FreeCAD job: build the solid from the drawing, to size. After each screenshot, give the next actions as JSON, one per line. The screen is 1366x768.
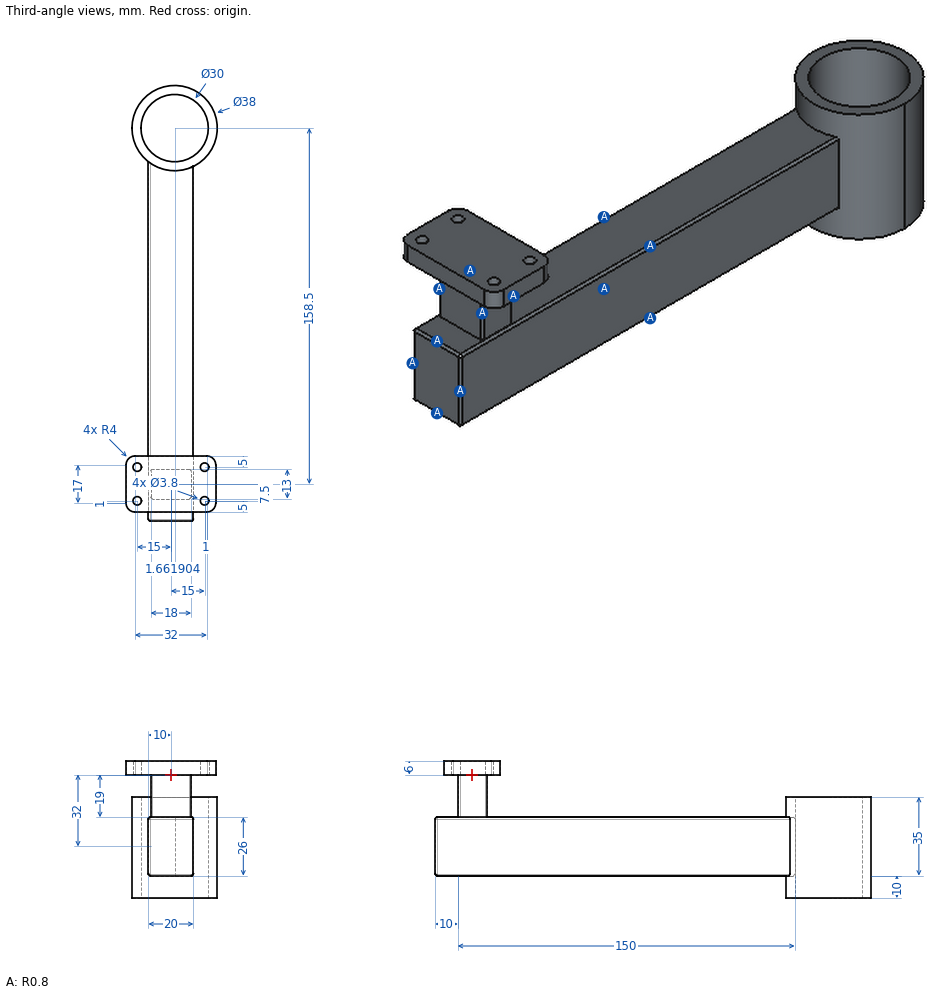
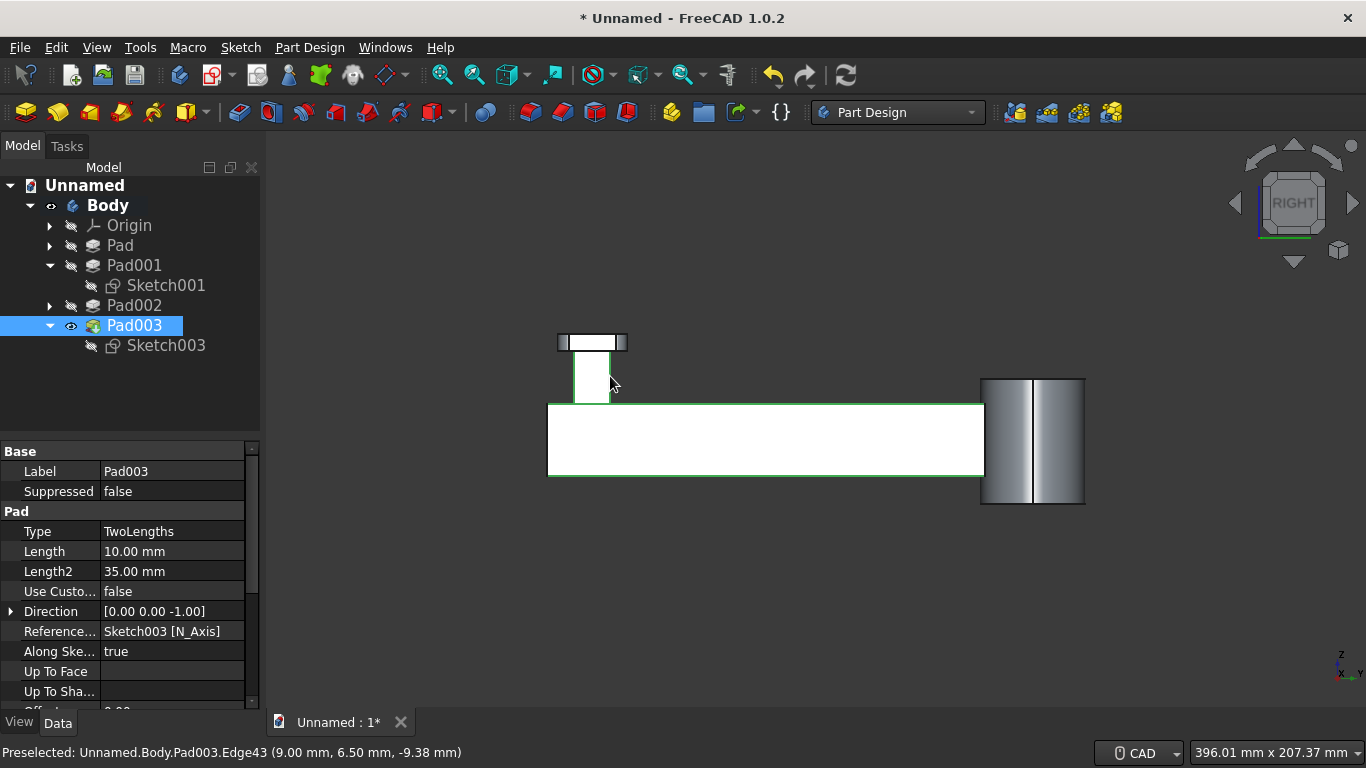
{"action": "key", "text": "5"}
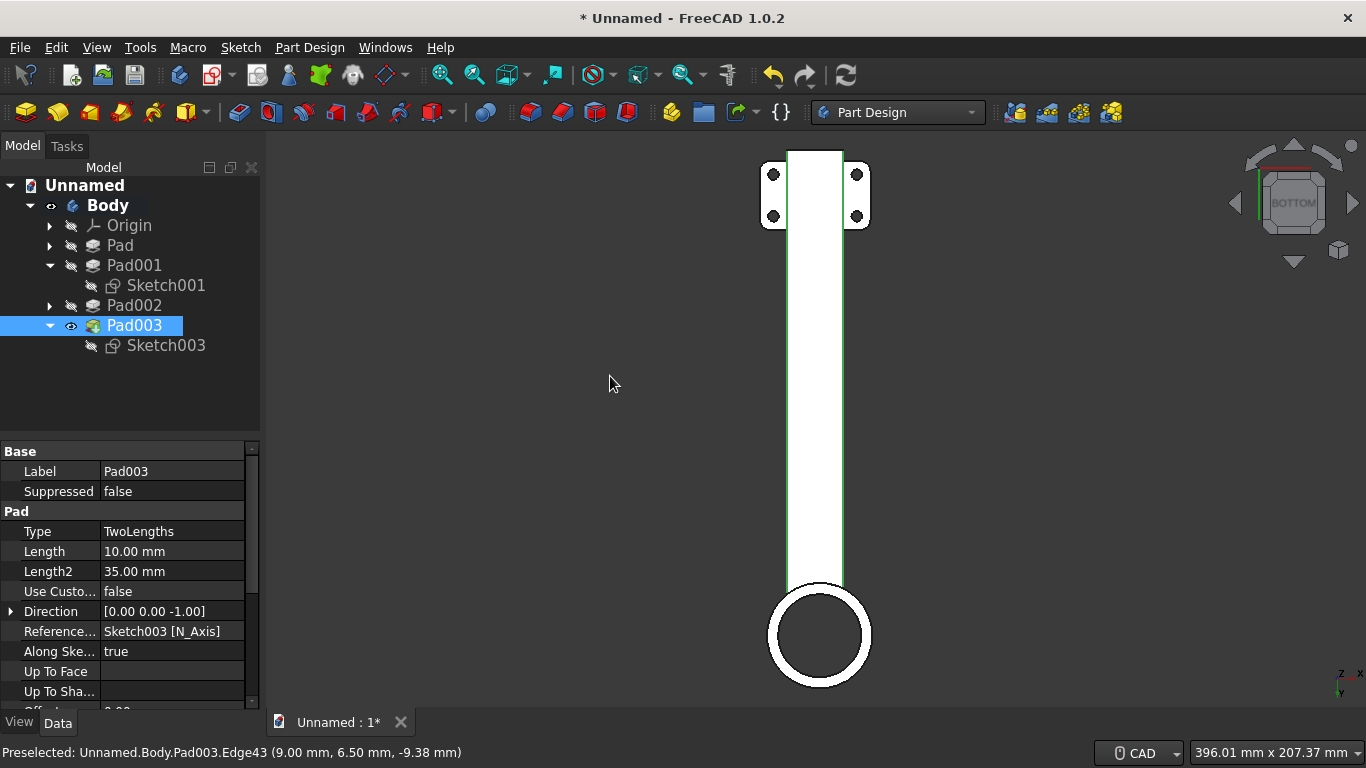
{"action": "key", "text": "4"}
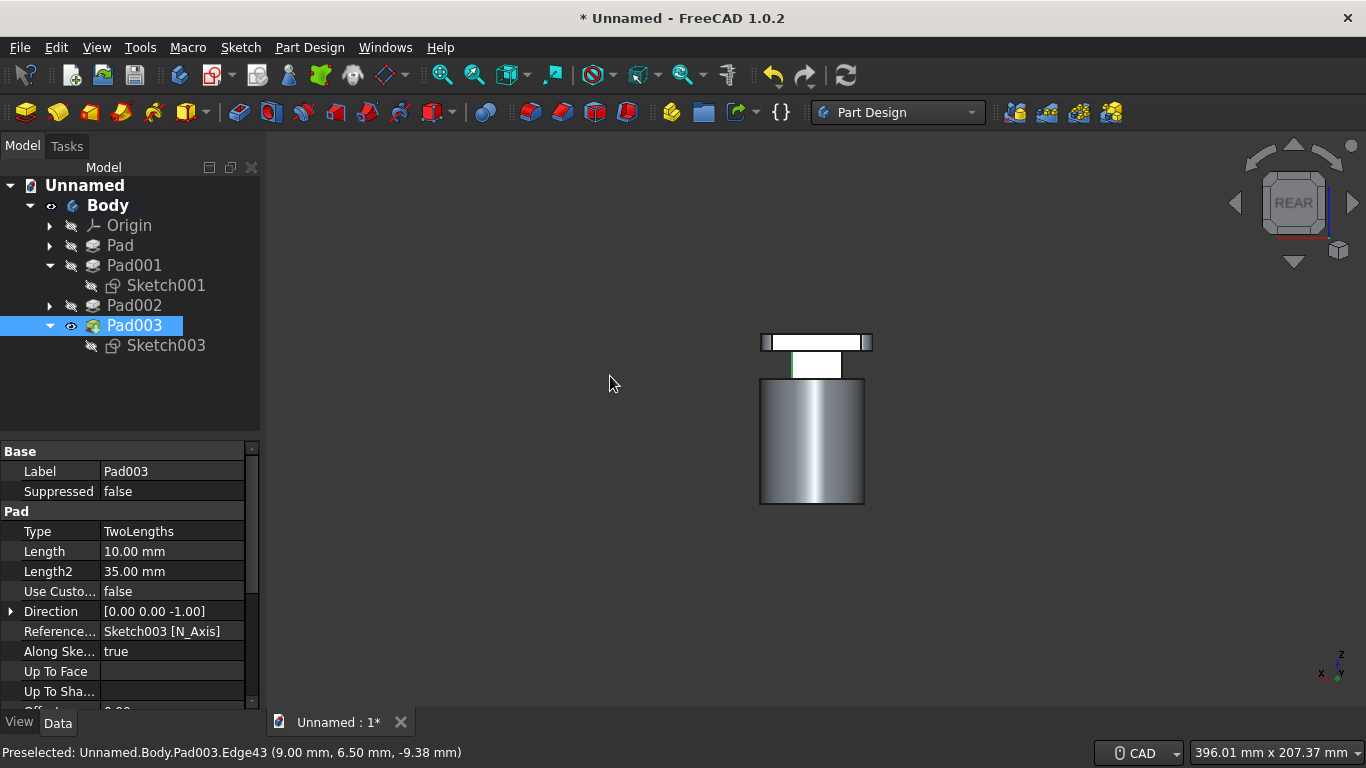
{"action": "left_click", "coordinate": [444, 76]}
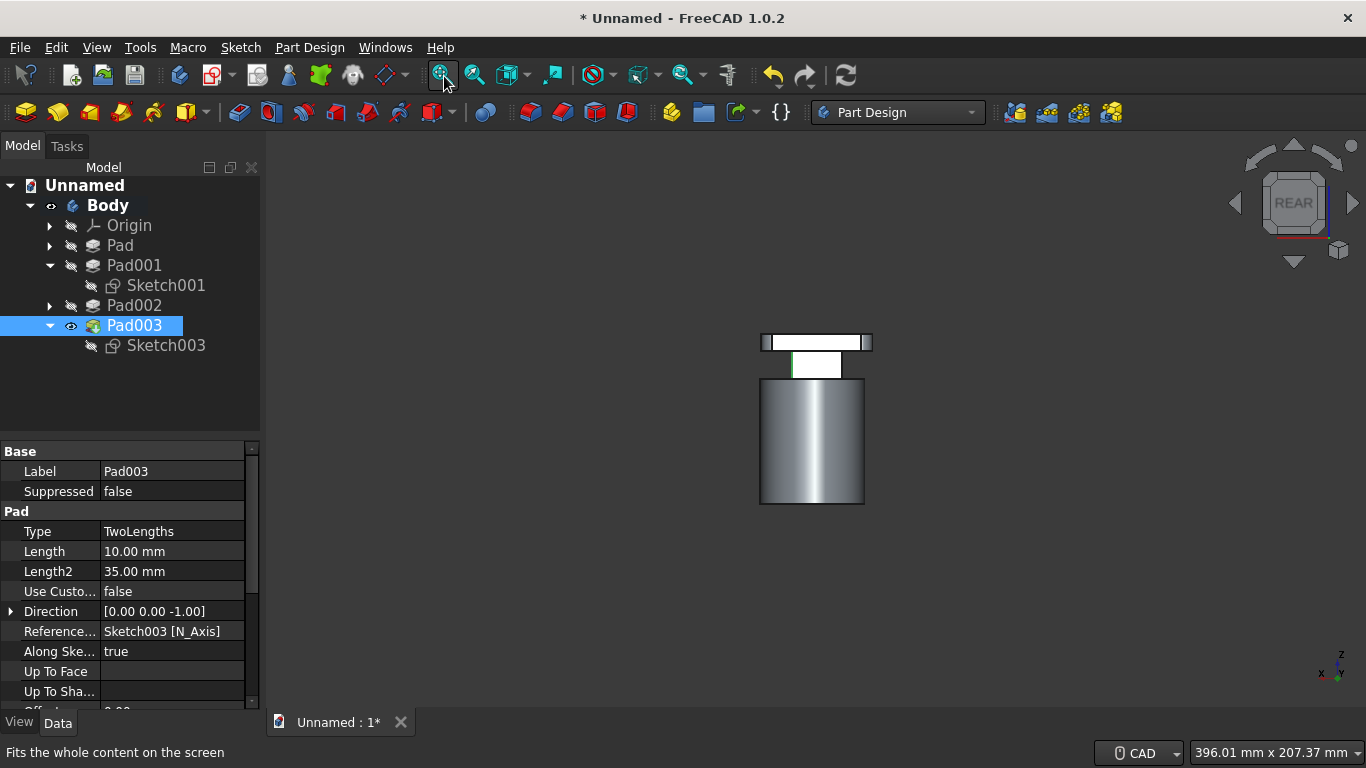
{"action": "left_click", "coordinate": [842, 371], "text": "ctrl"}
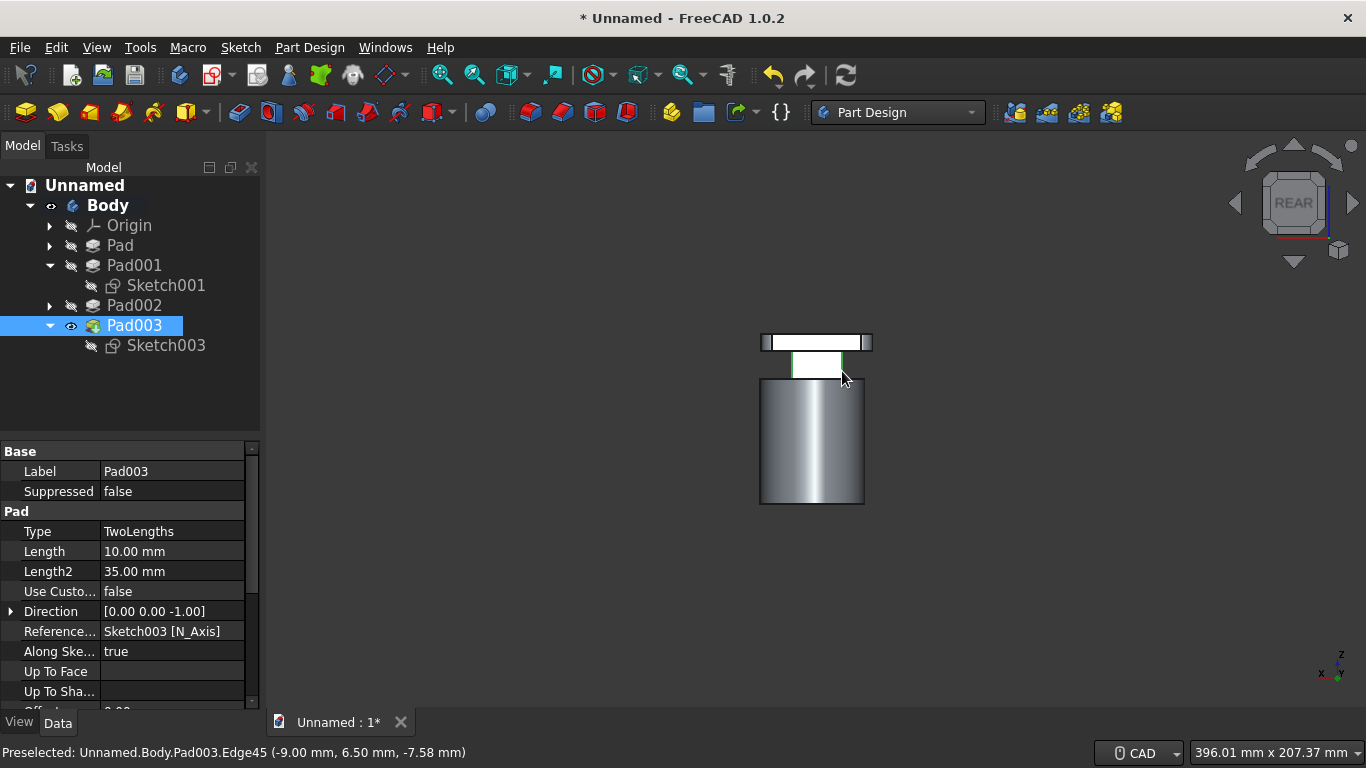
{"action": "left_click", "coordinate": [532, 112]}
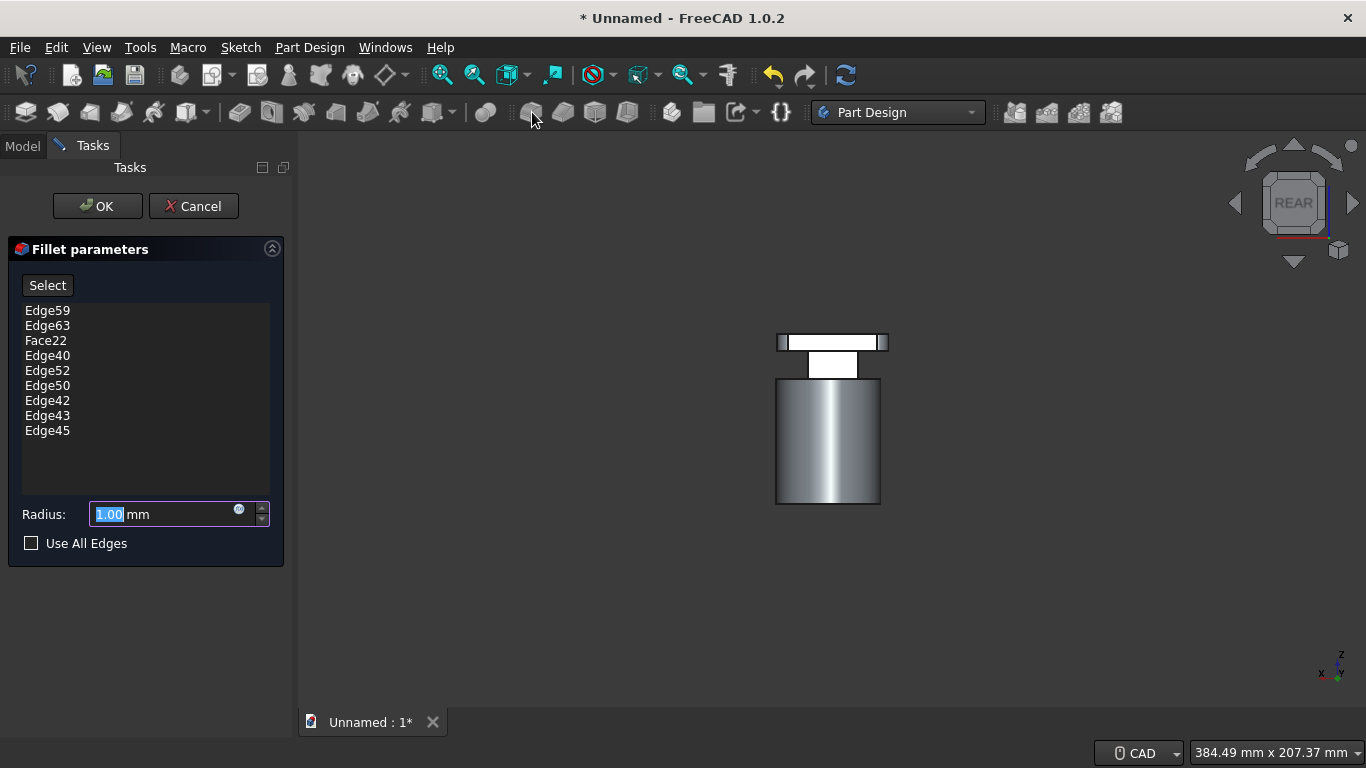
{"action": "type", "text": "0.8"}
{"action": "key", "text": "Tab"}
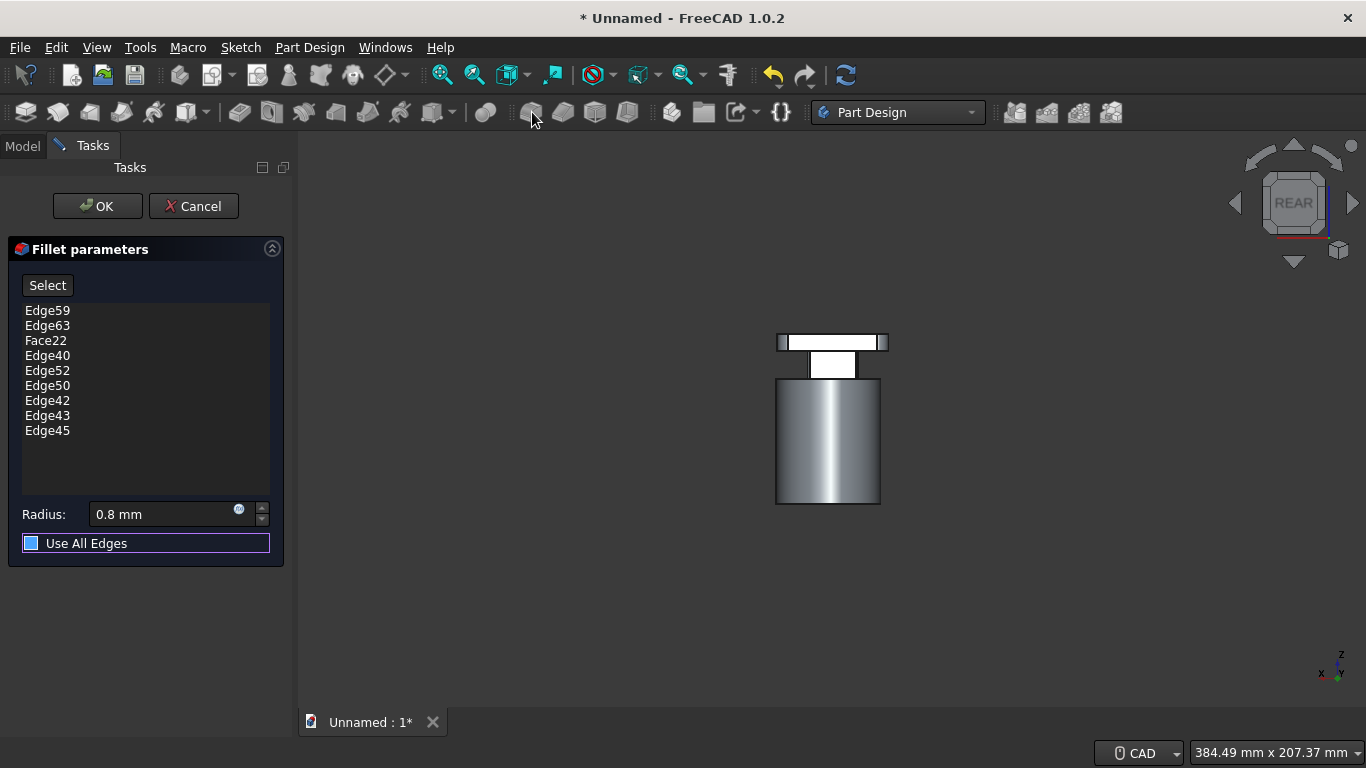
{"action": "left_click", "coordinate": [98, 206]}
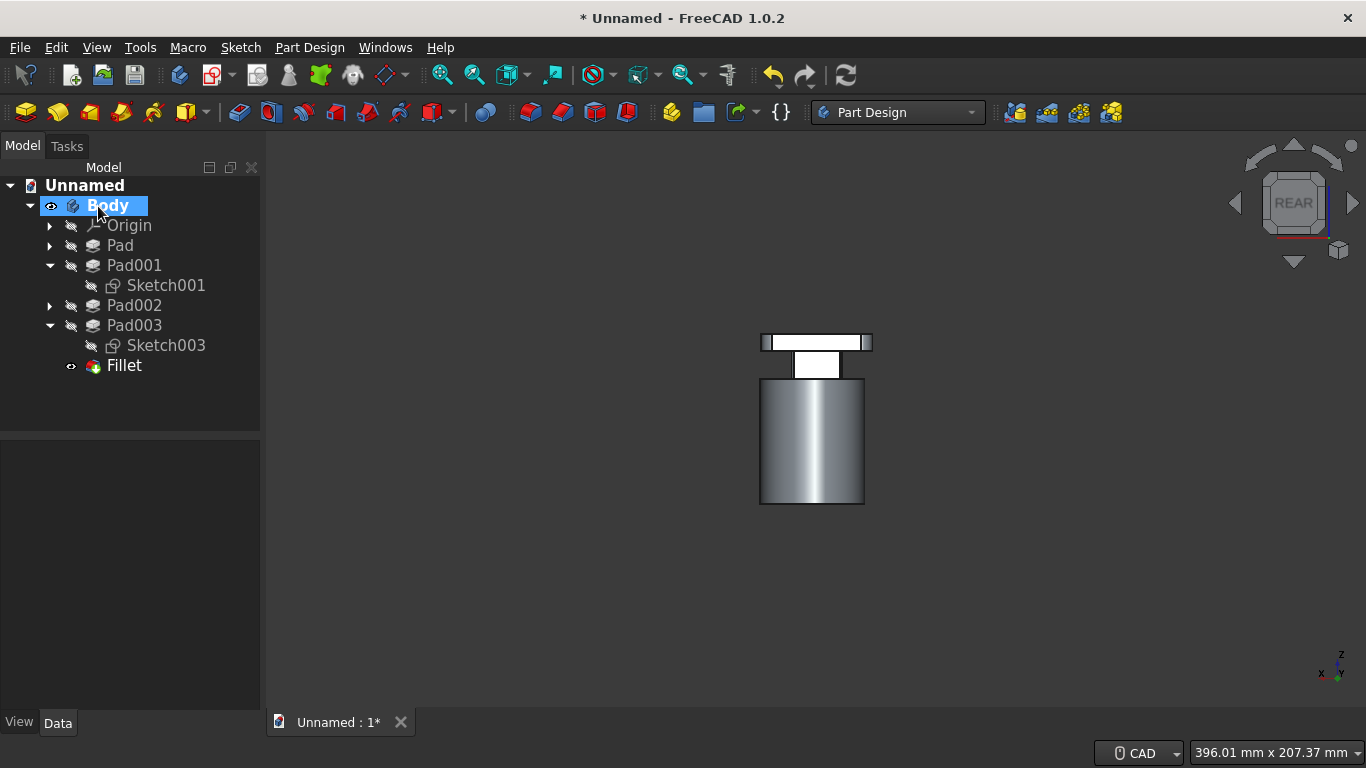
{"action": "key", "text": "0"}